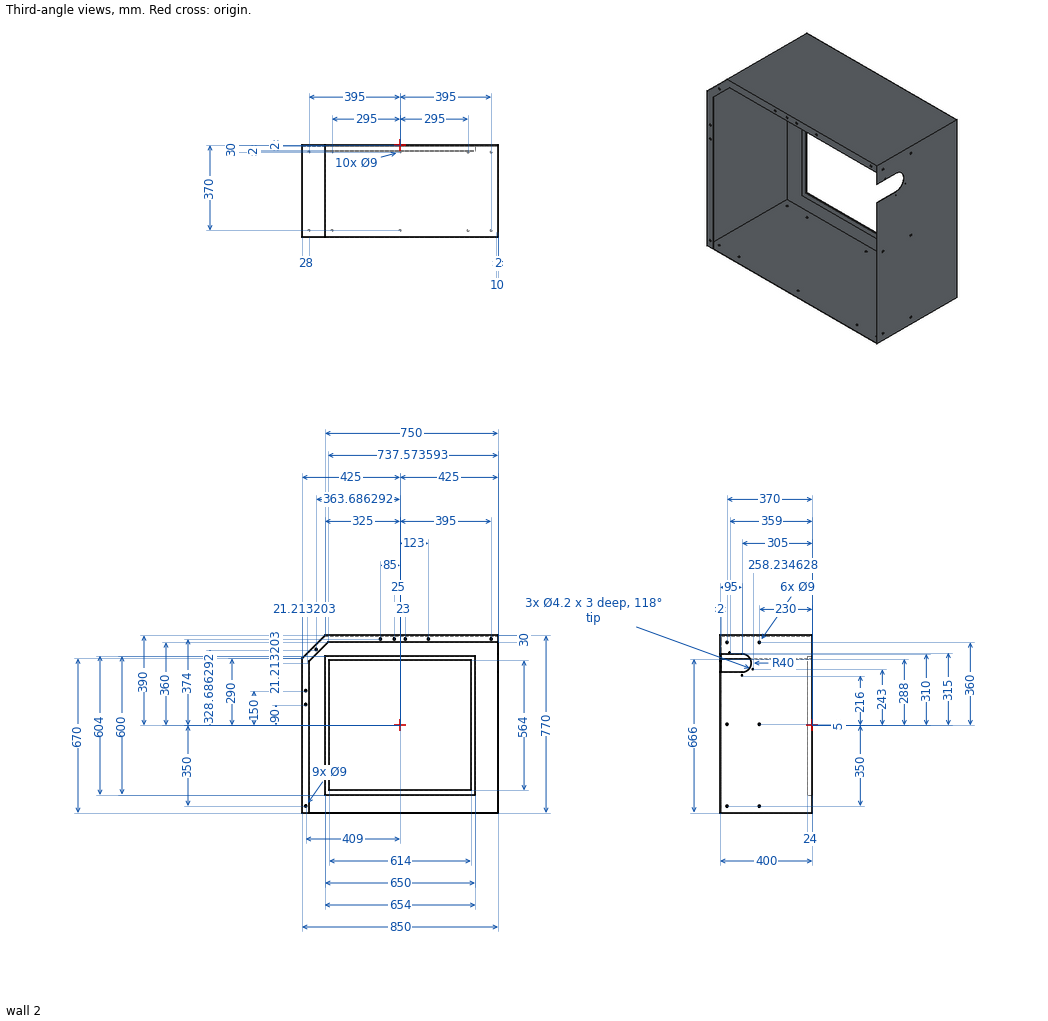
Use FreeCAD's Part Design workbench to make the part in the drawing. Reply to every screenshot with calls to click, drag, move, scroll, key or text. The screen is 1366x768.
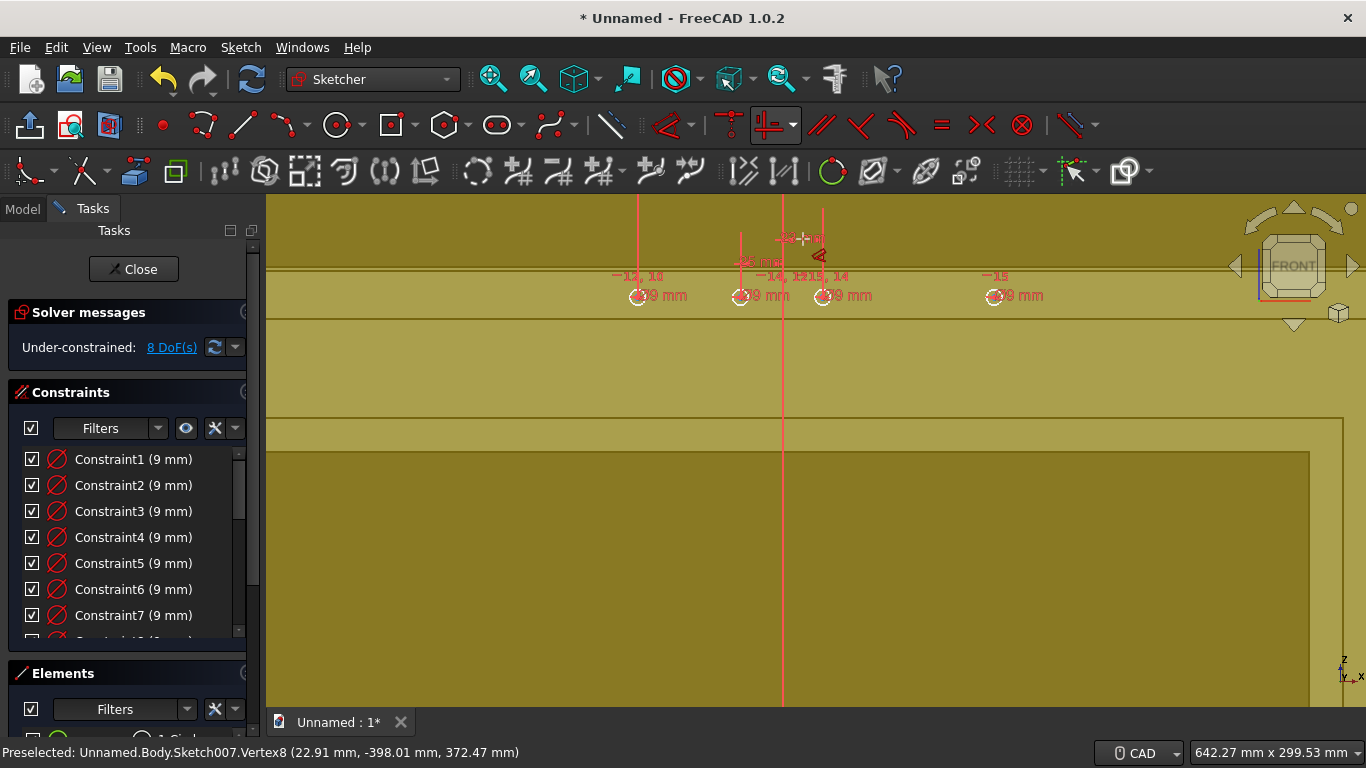
scroll(740, 299, down, 7)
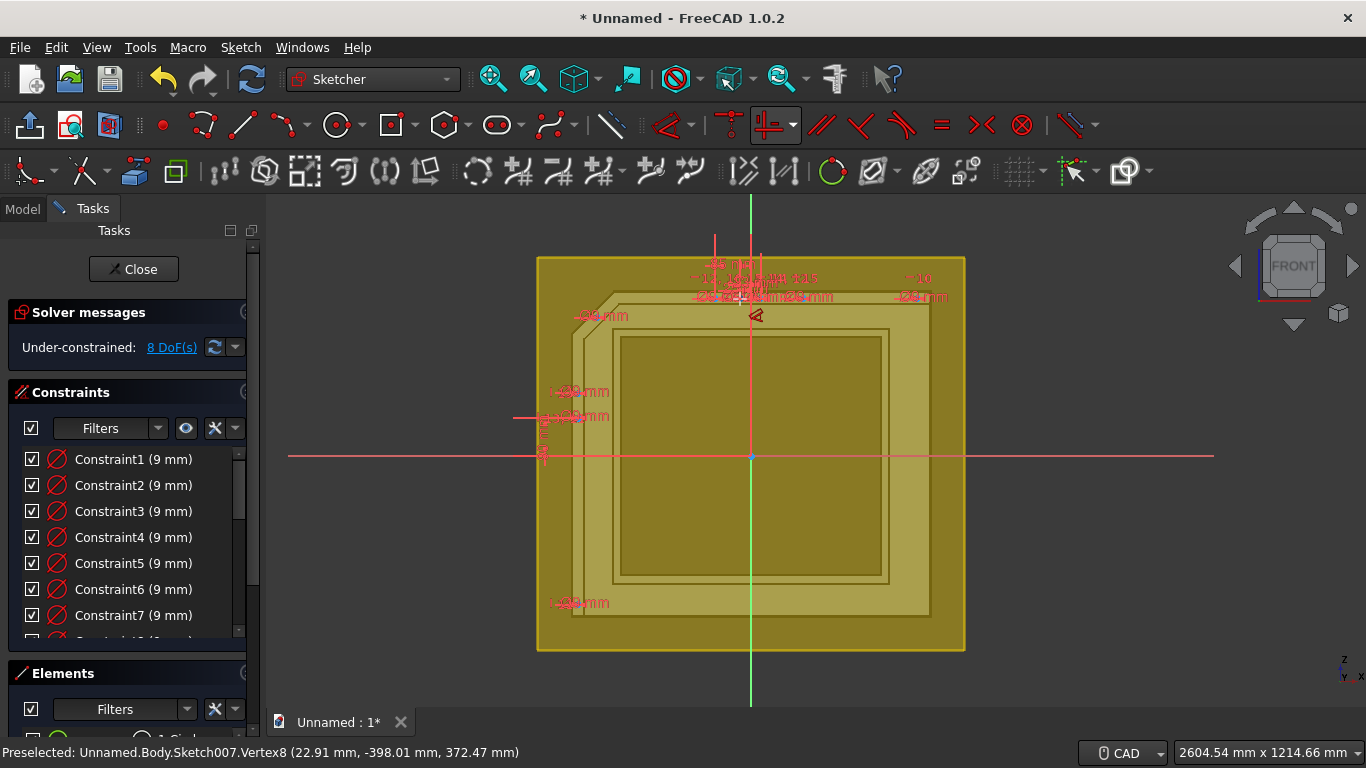
click(579, 605)
click(665, 639)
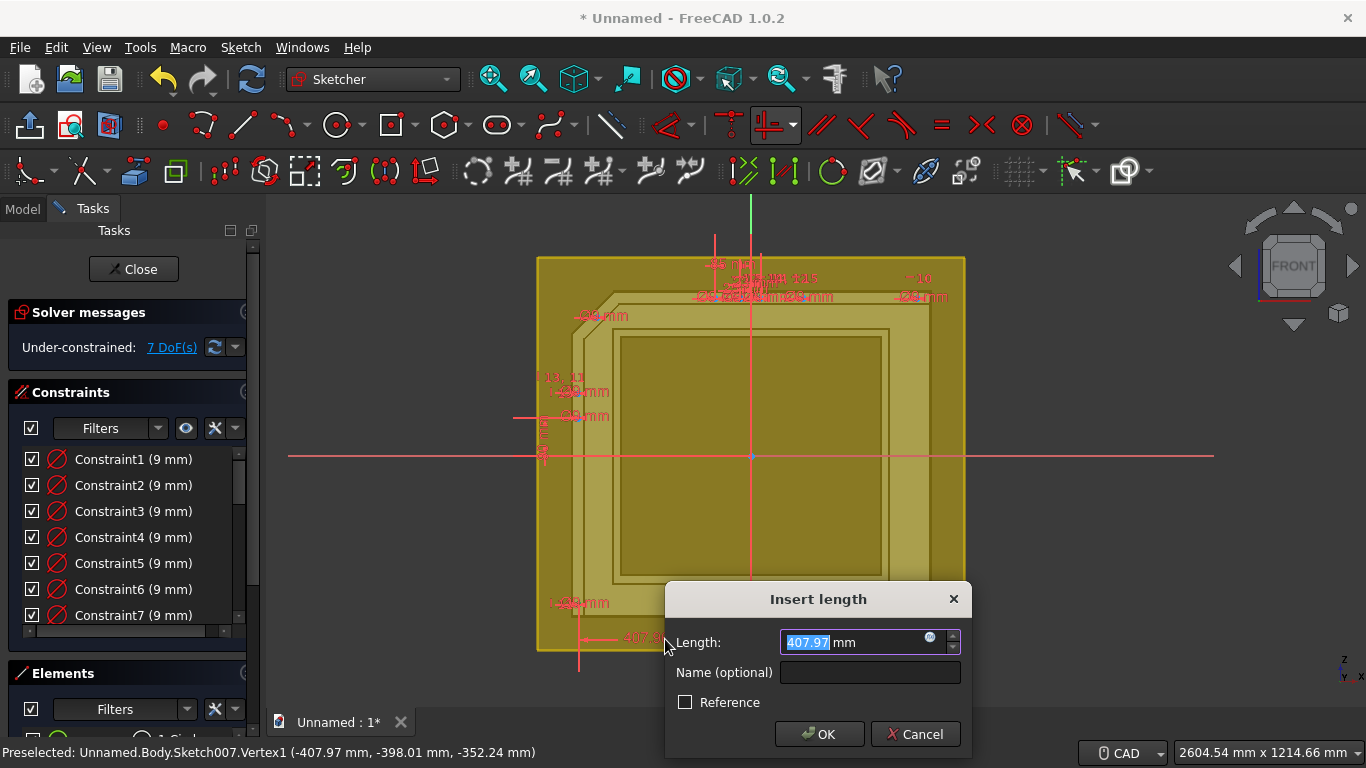
text(409)
key(Return)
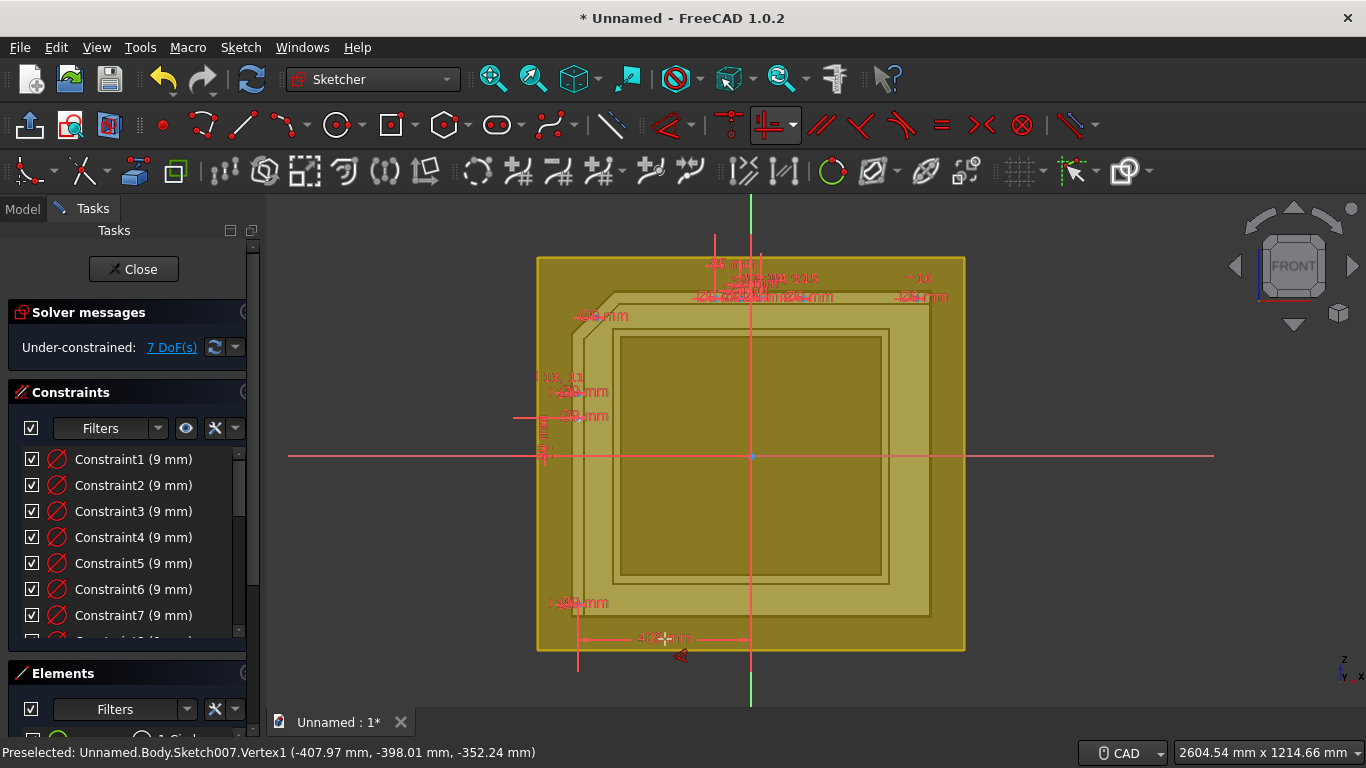
click(578, 605)
click(544, 530)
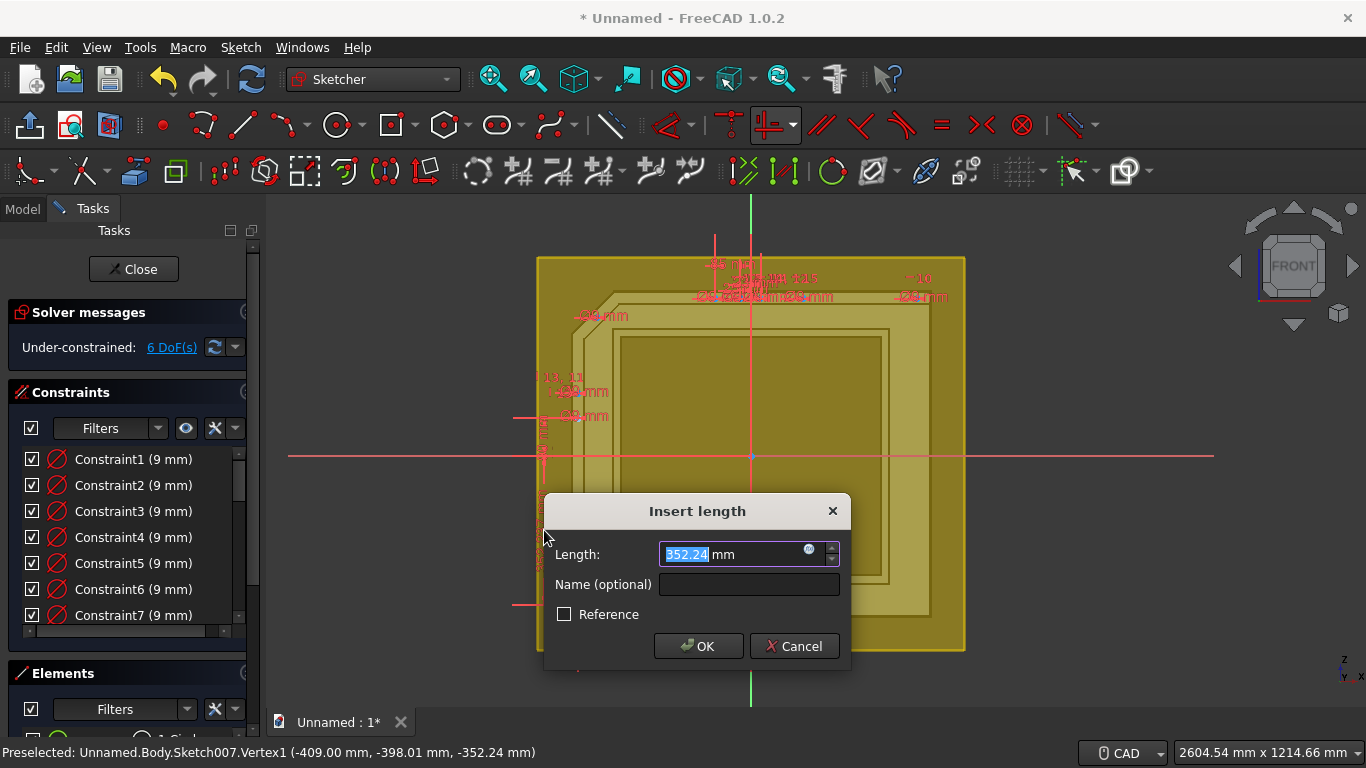
text(350)
key(Return)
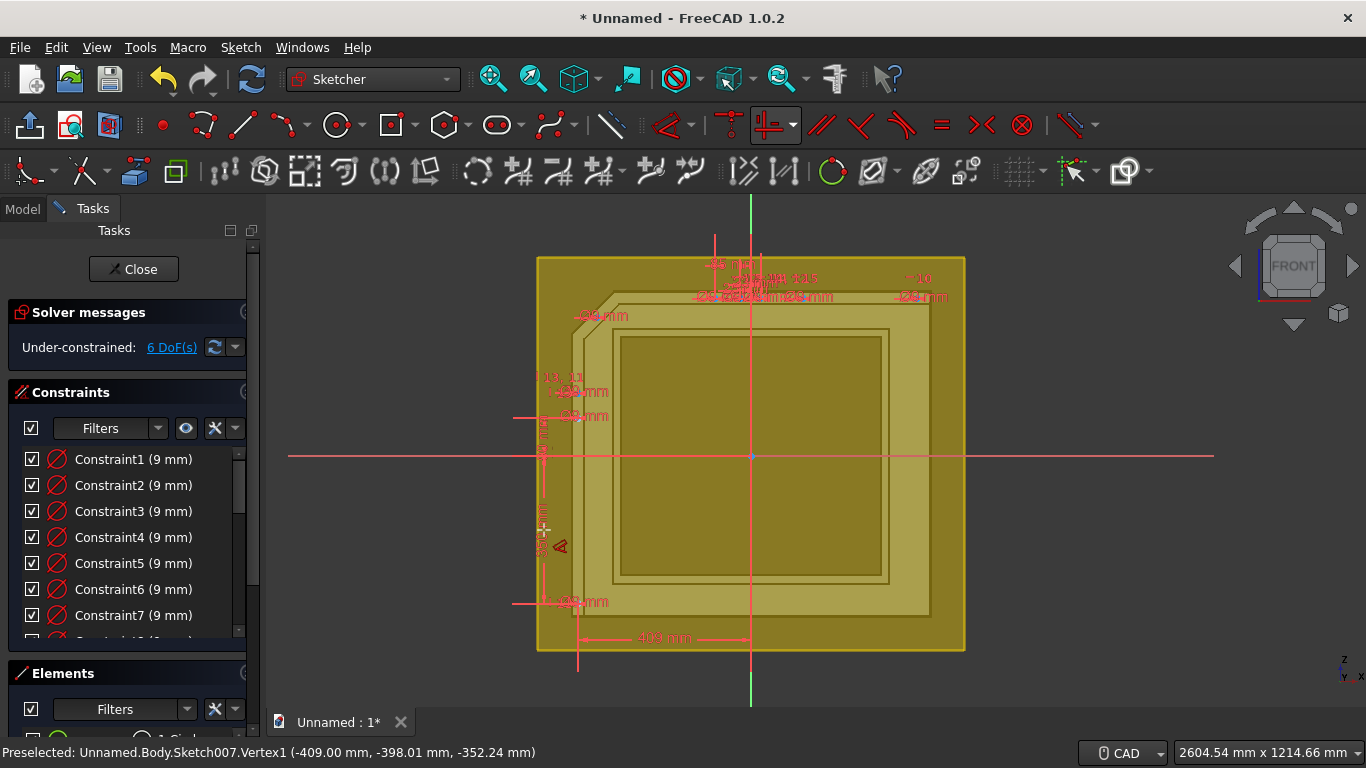
click(715, 299)
click(681, 377)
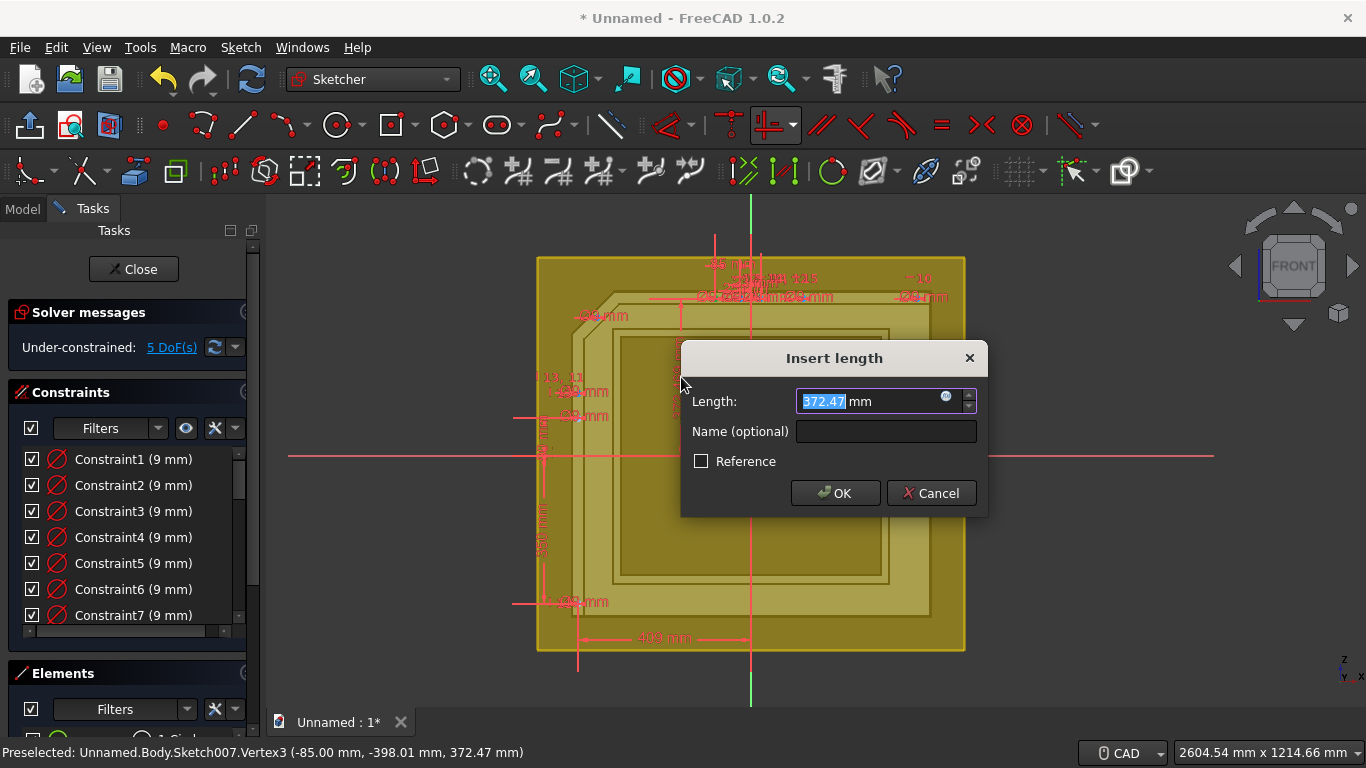
text(374)
key(Return)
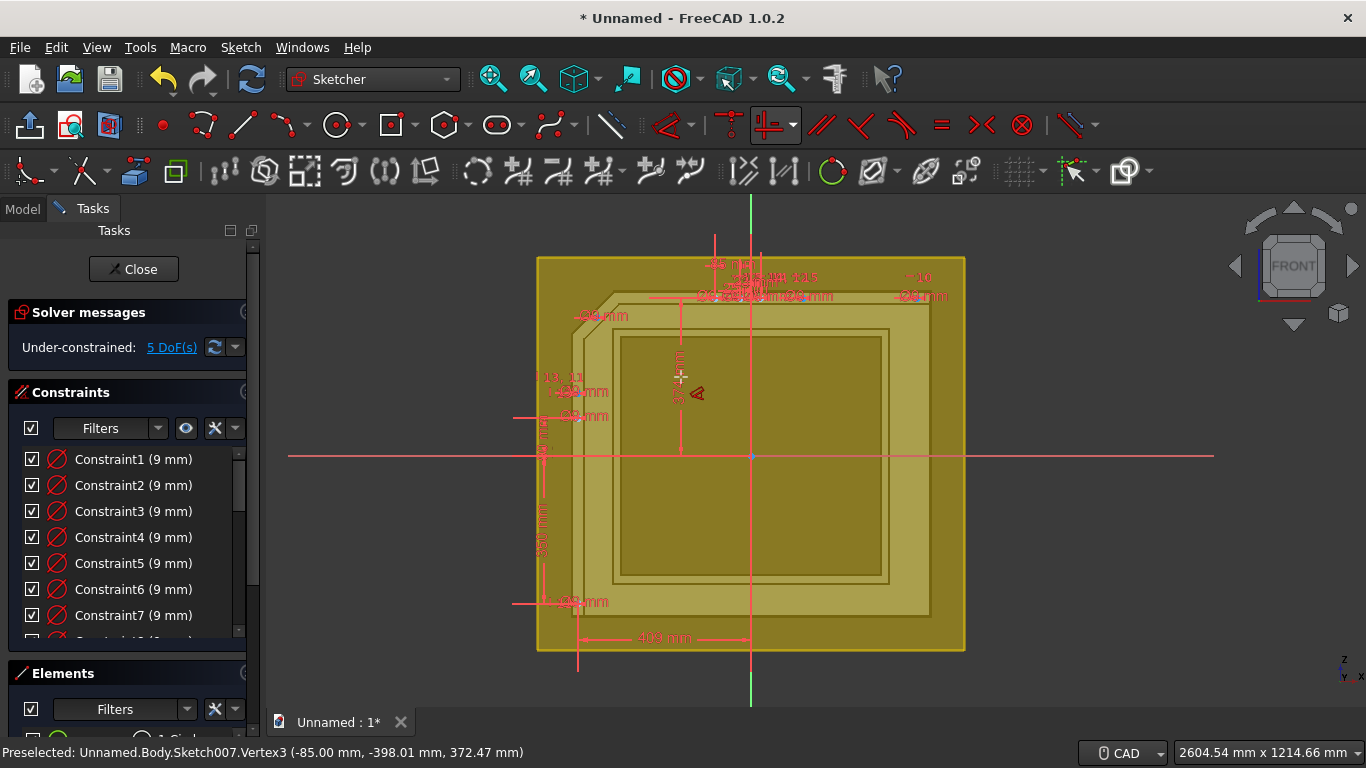
click(918, 298)
click(834, 264)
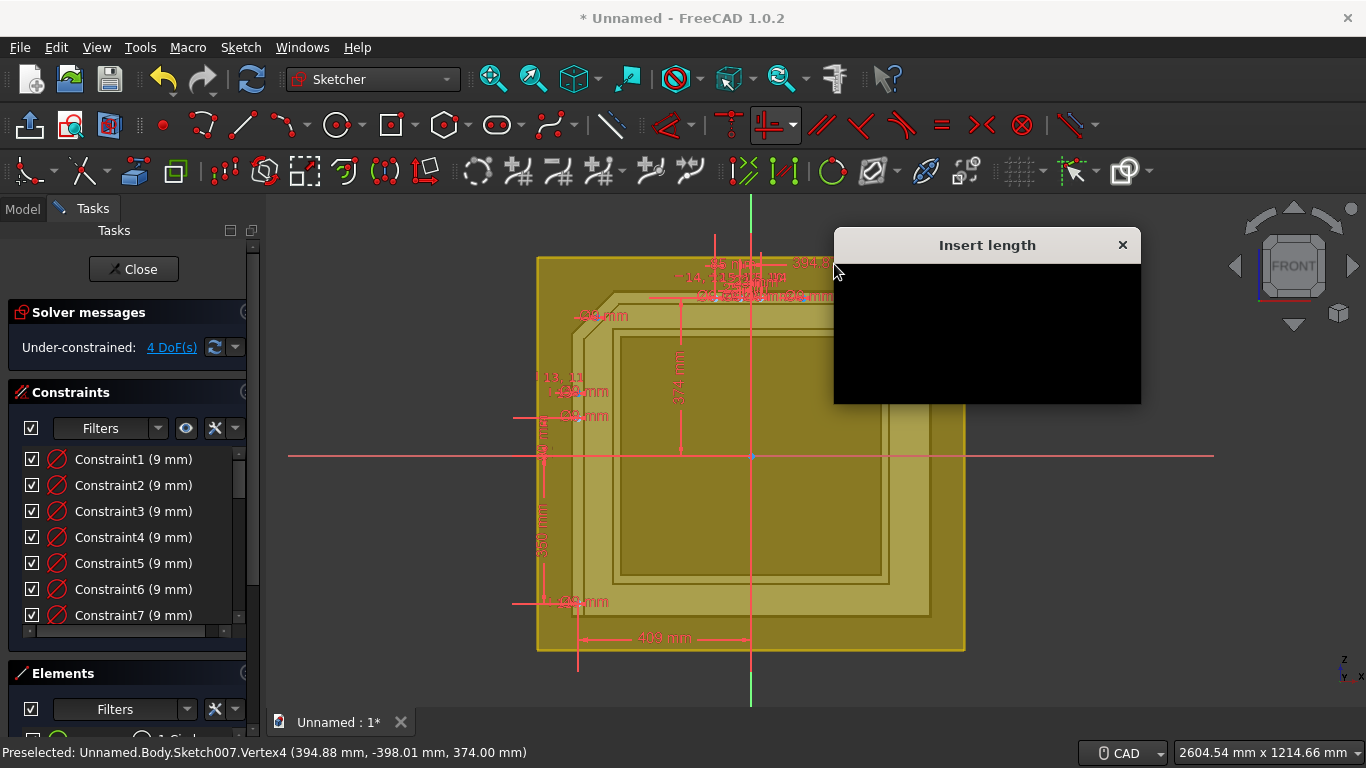
text(395)
key(Return)